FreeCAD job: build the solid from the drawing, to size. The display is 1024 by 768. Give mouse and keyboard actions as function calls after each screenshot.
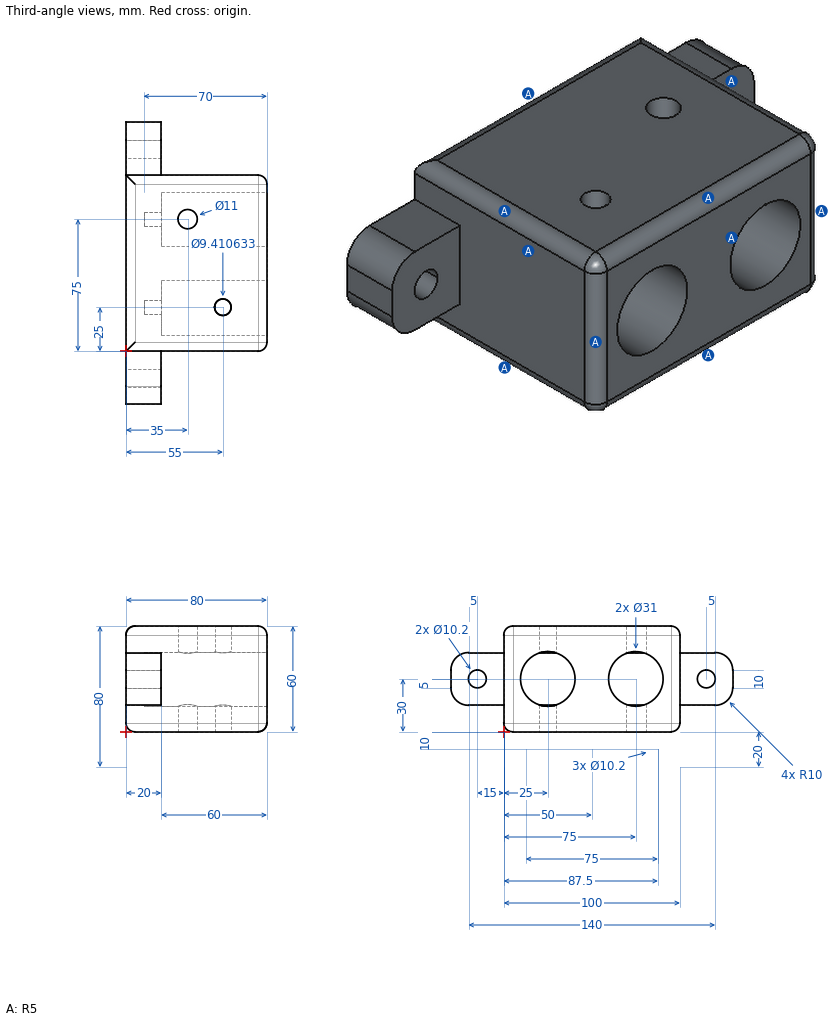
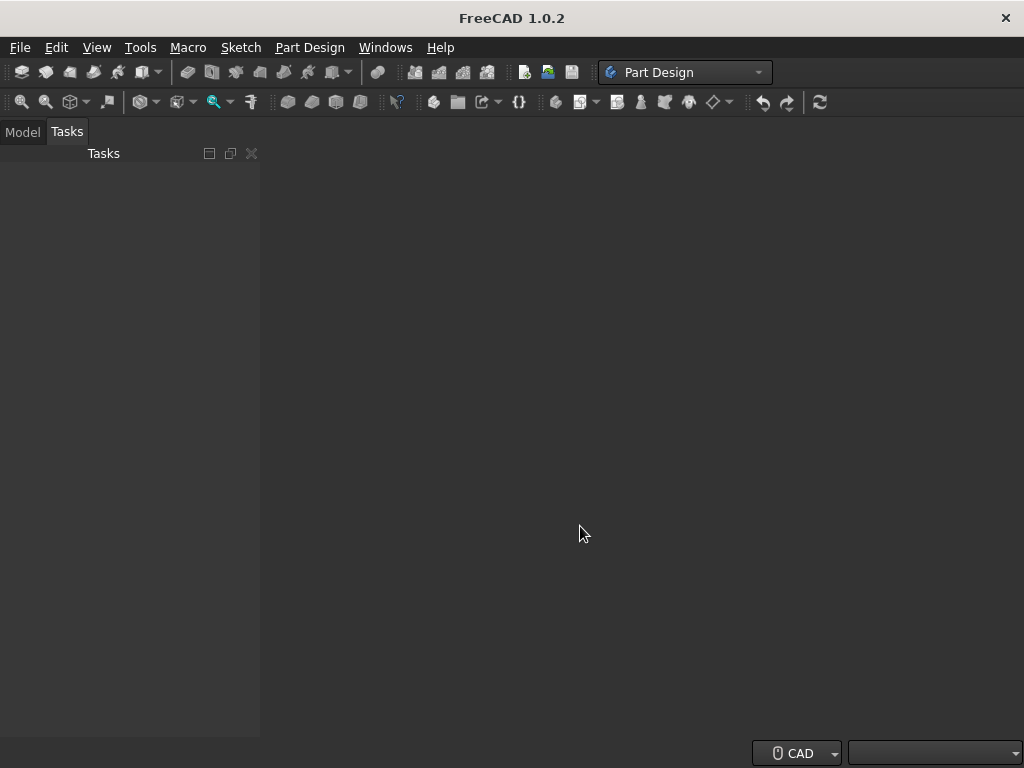
key(ctrl+n)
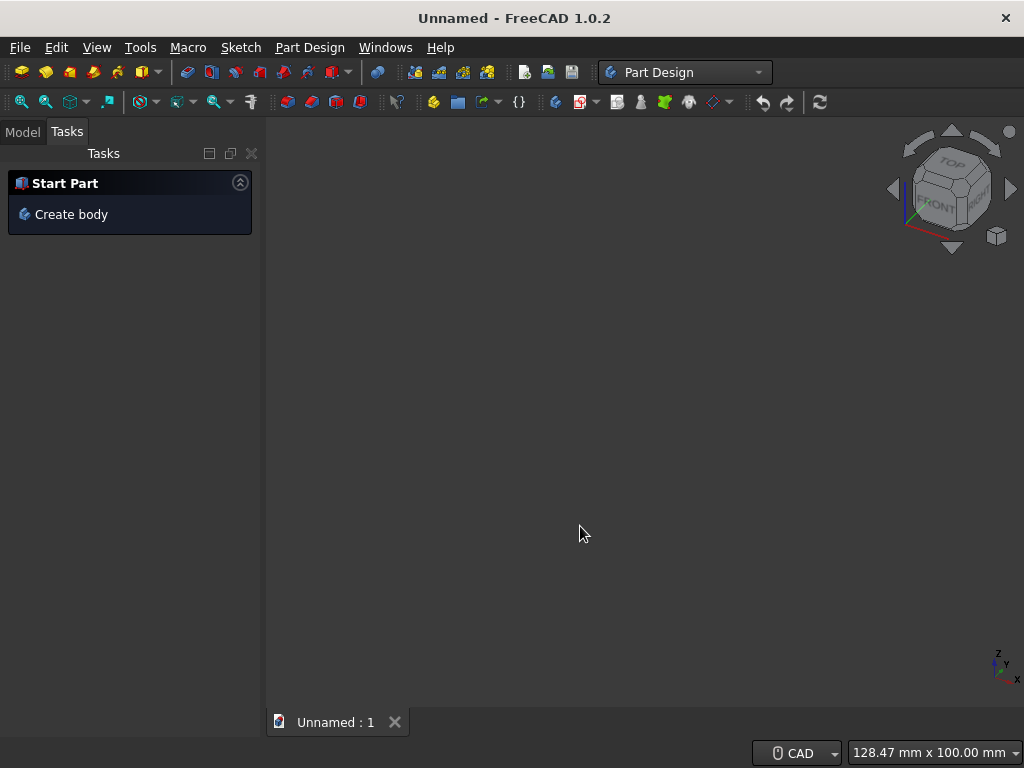
click(580, 102)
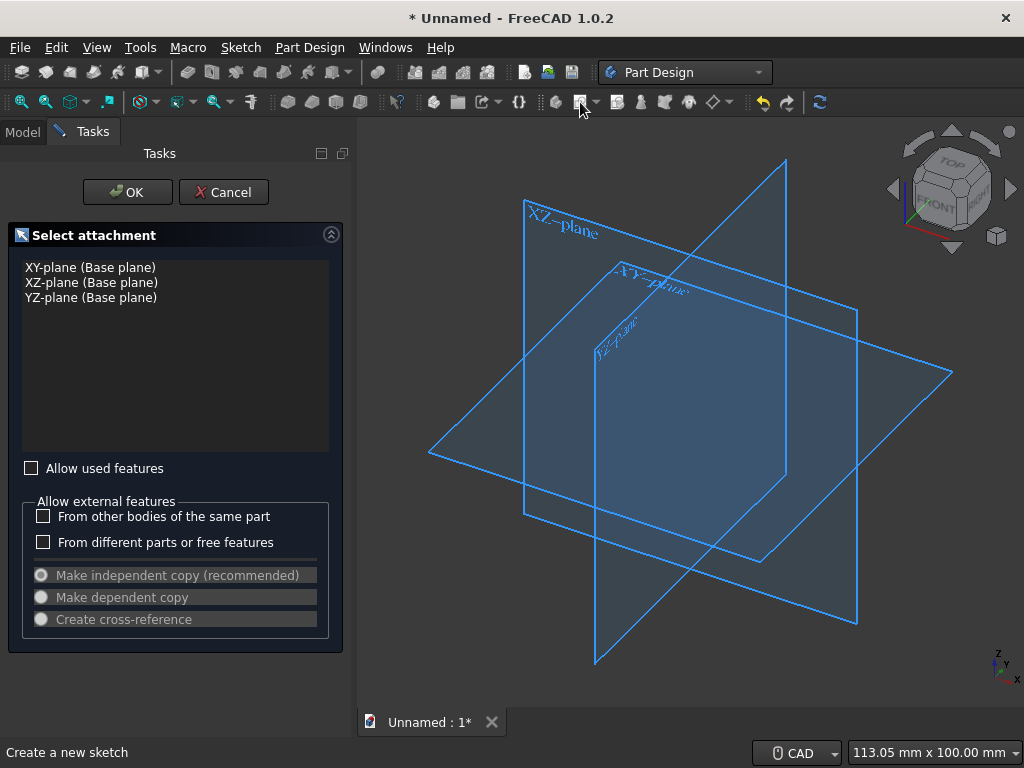
click(82, 282)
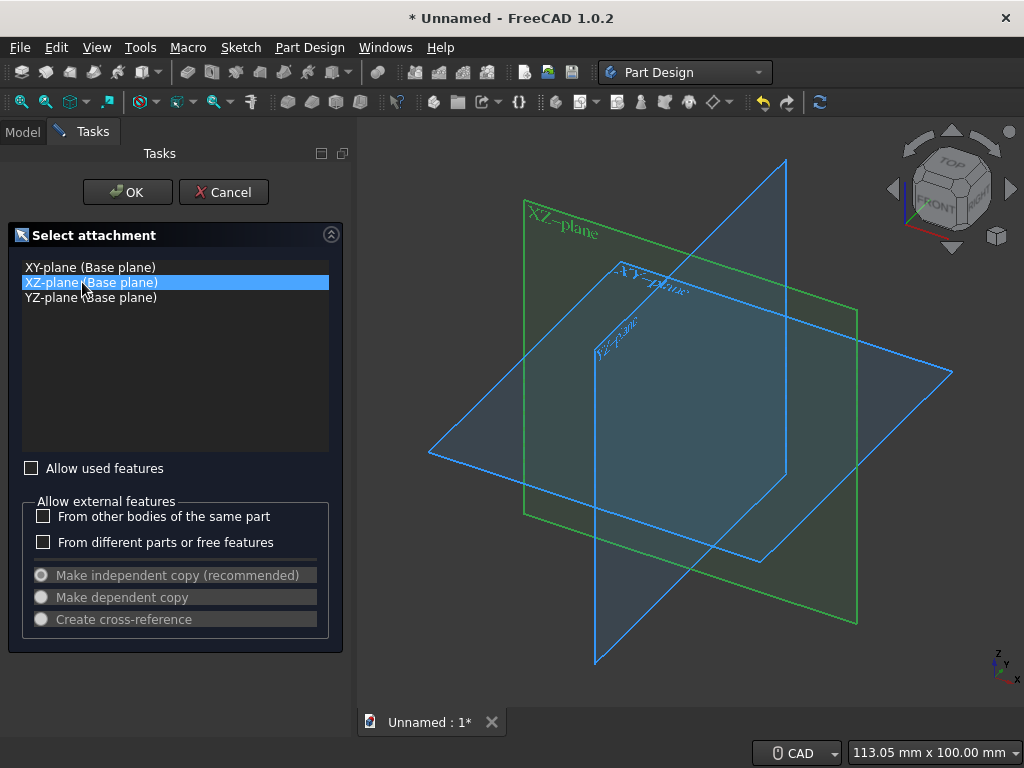
click(128, 192)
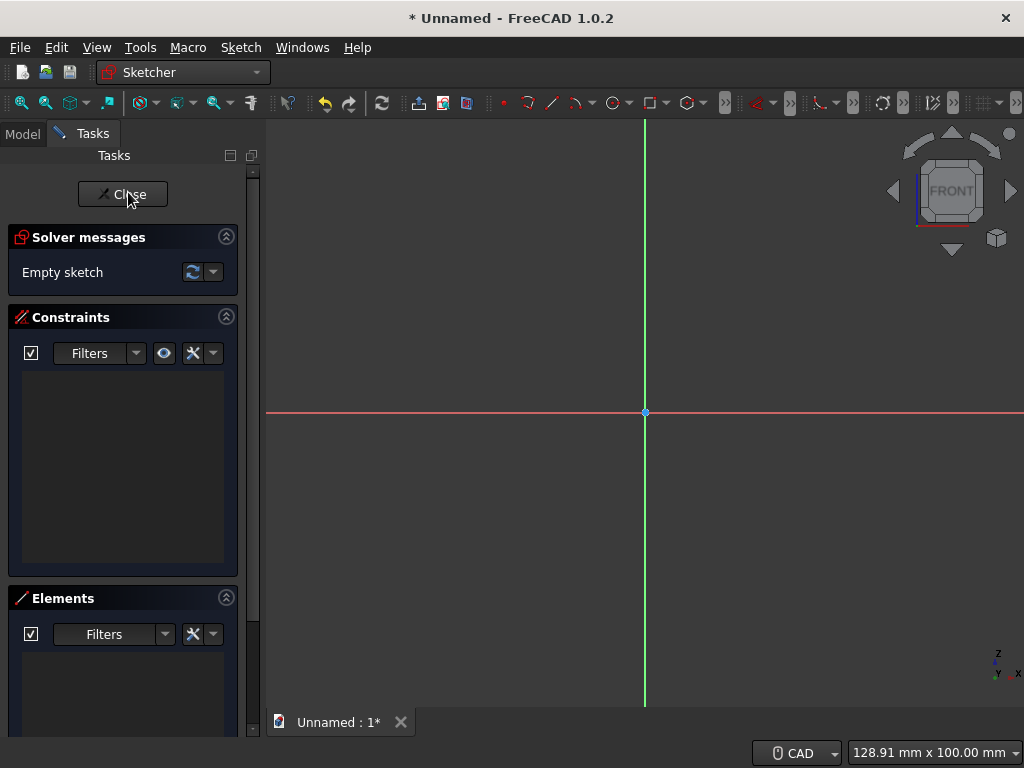
scroll(294, 556, down, 3)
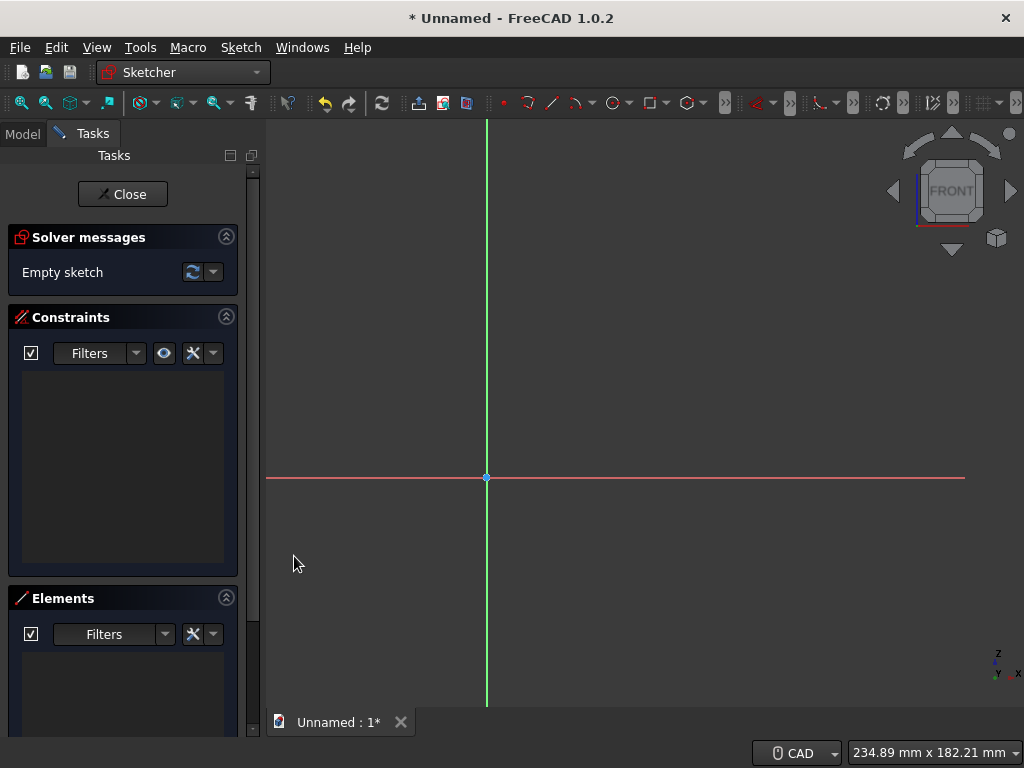
scroll(695, 414, up, 2)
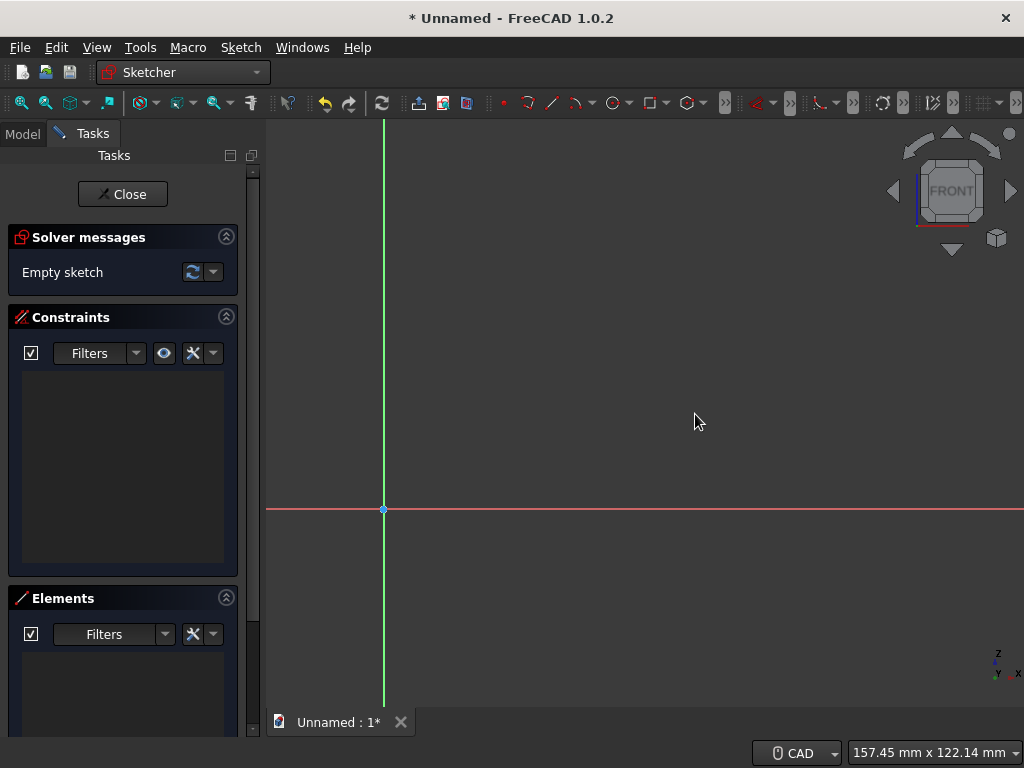
click(528, 104)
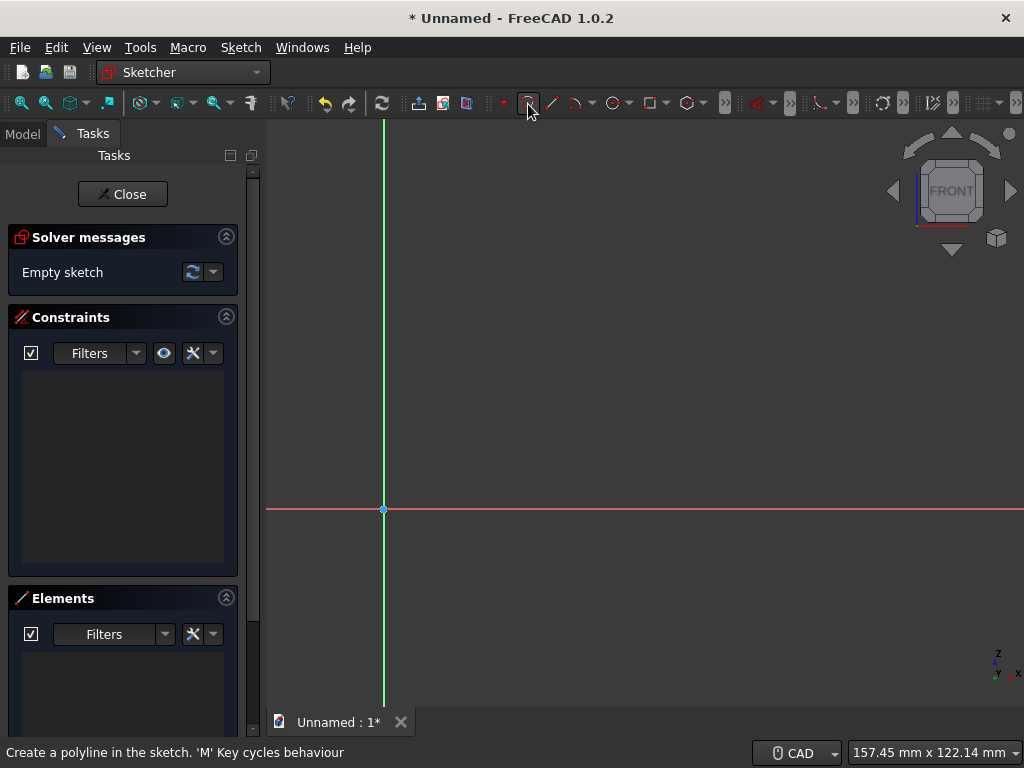
click(384, 605)
click(393, 220)
click(769, 220)
click(769, 509)
click(480, 500)
click(480, 605)
click(384, 606)
key(Escape)
key(Escape)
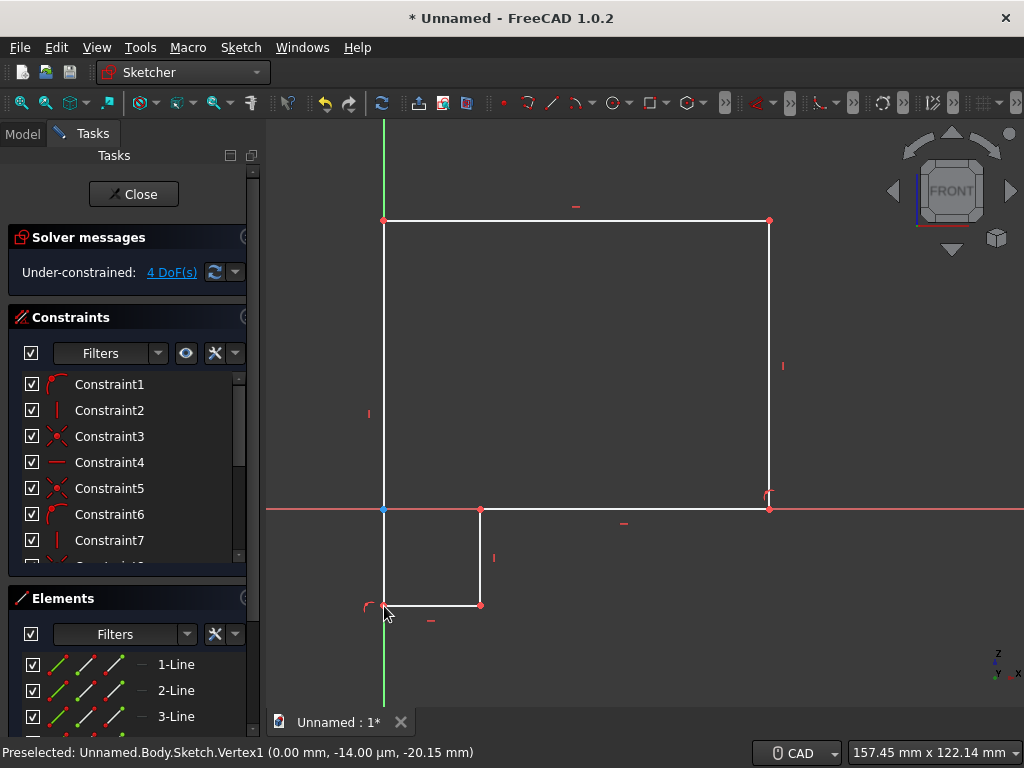
click(384, 490)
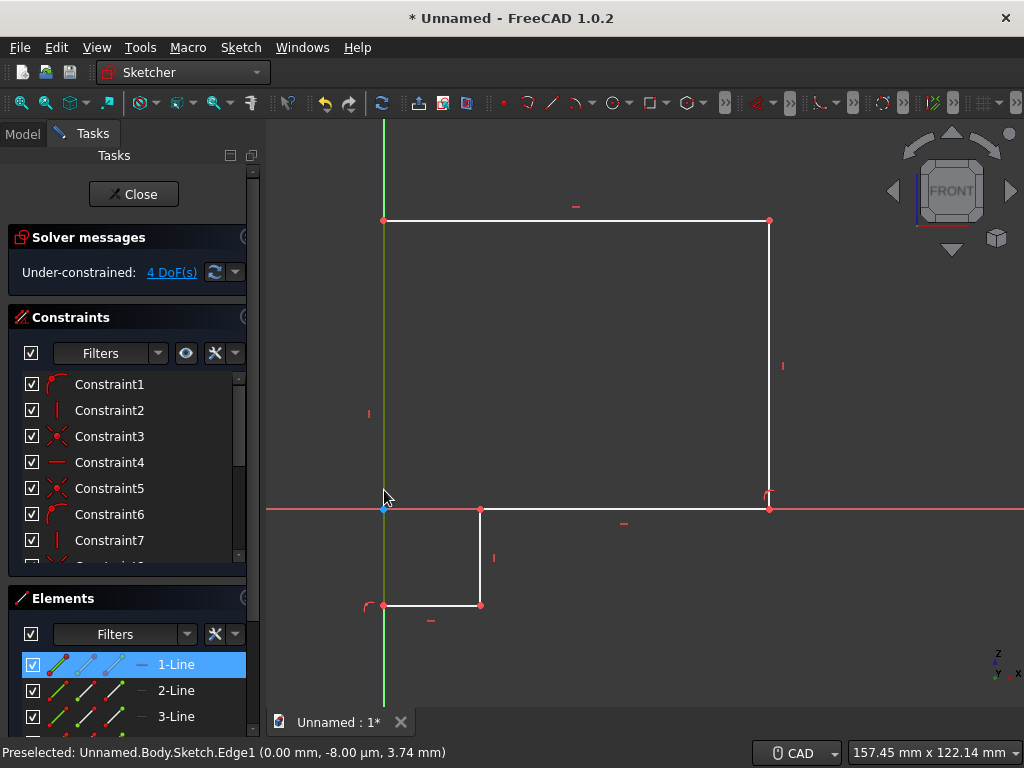
click(776, 104)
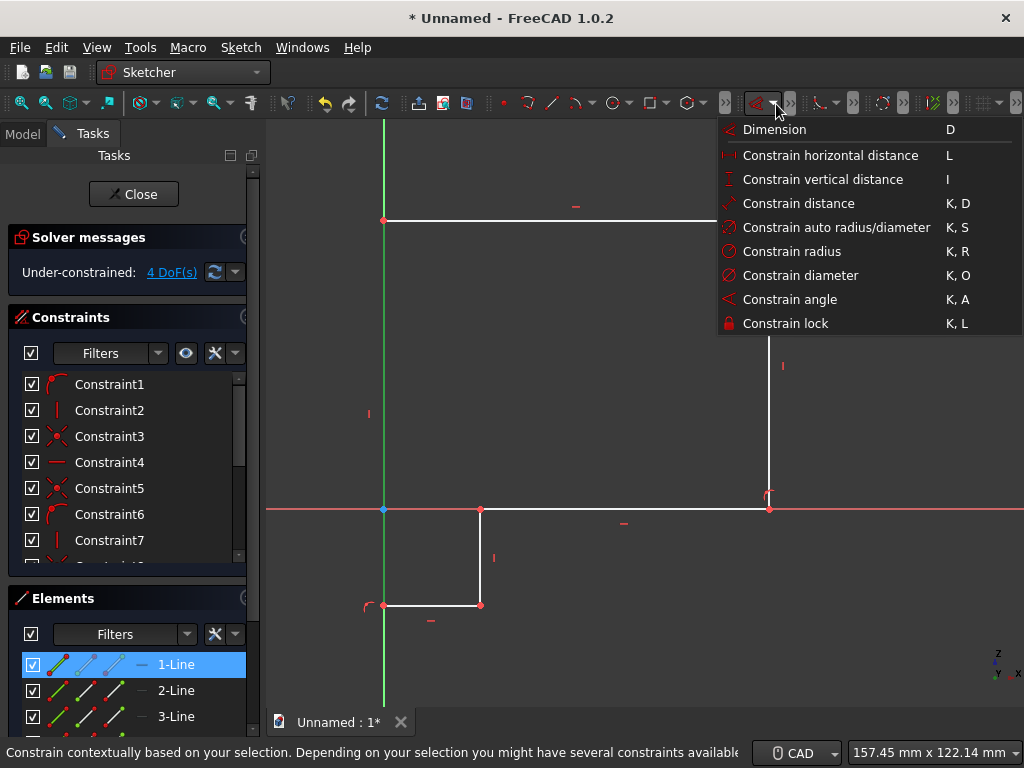
click(870, 179)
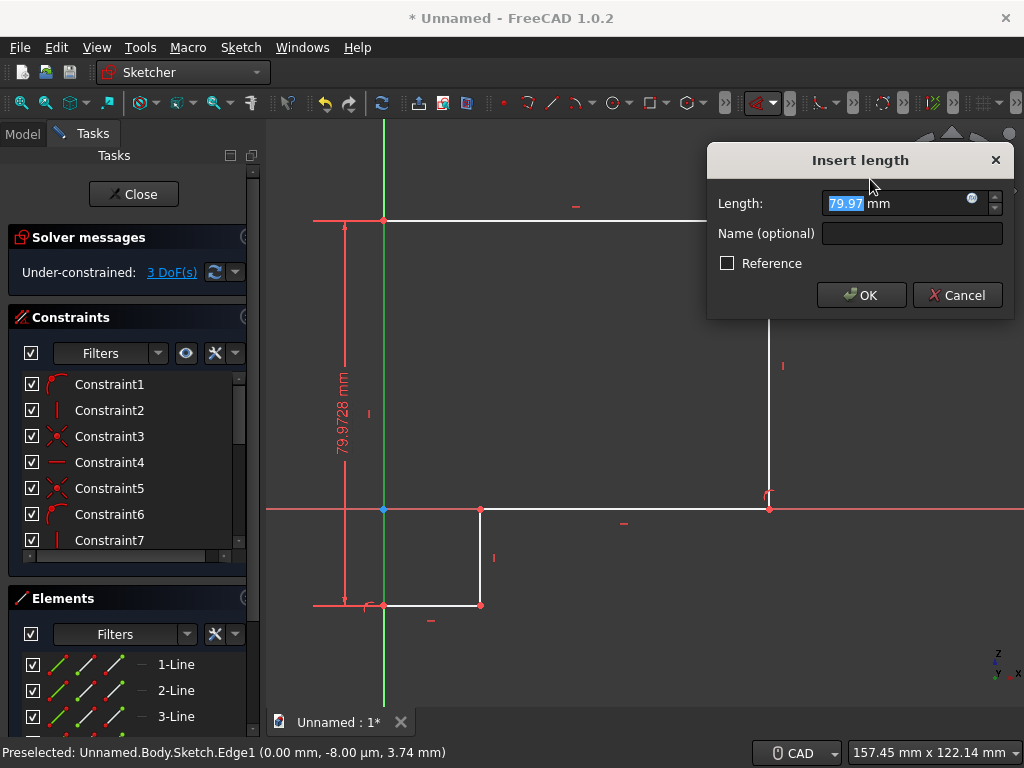
text(80)
key(Return)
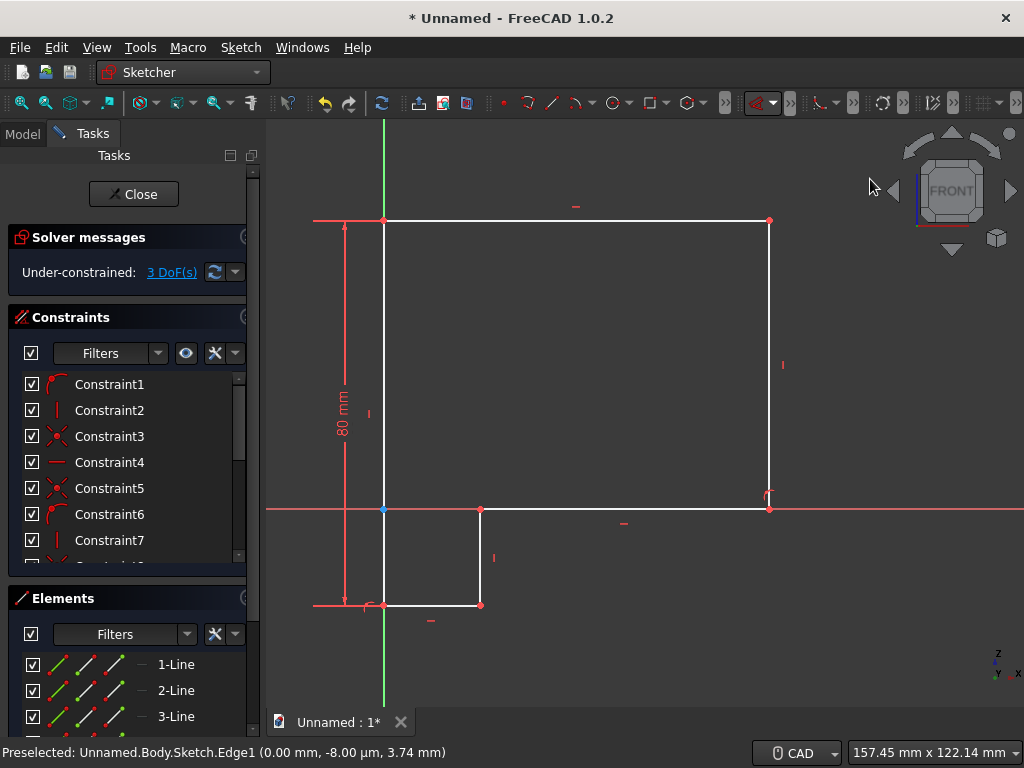
click(499, 221)